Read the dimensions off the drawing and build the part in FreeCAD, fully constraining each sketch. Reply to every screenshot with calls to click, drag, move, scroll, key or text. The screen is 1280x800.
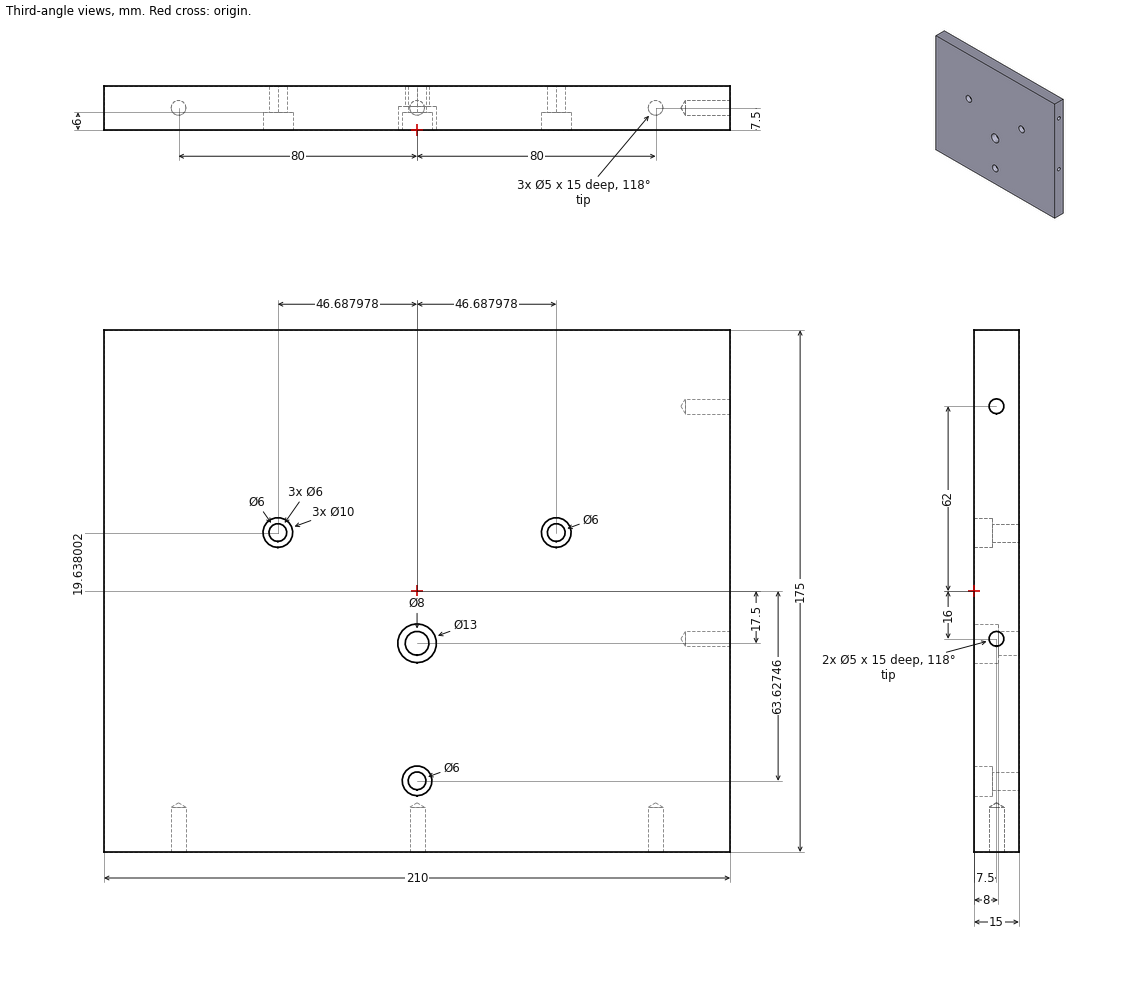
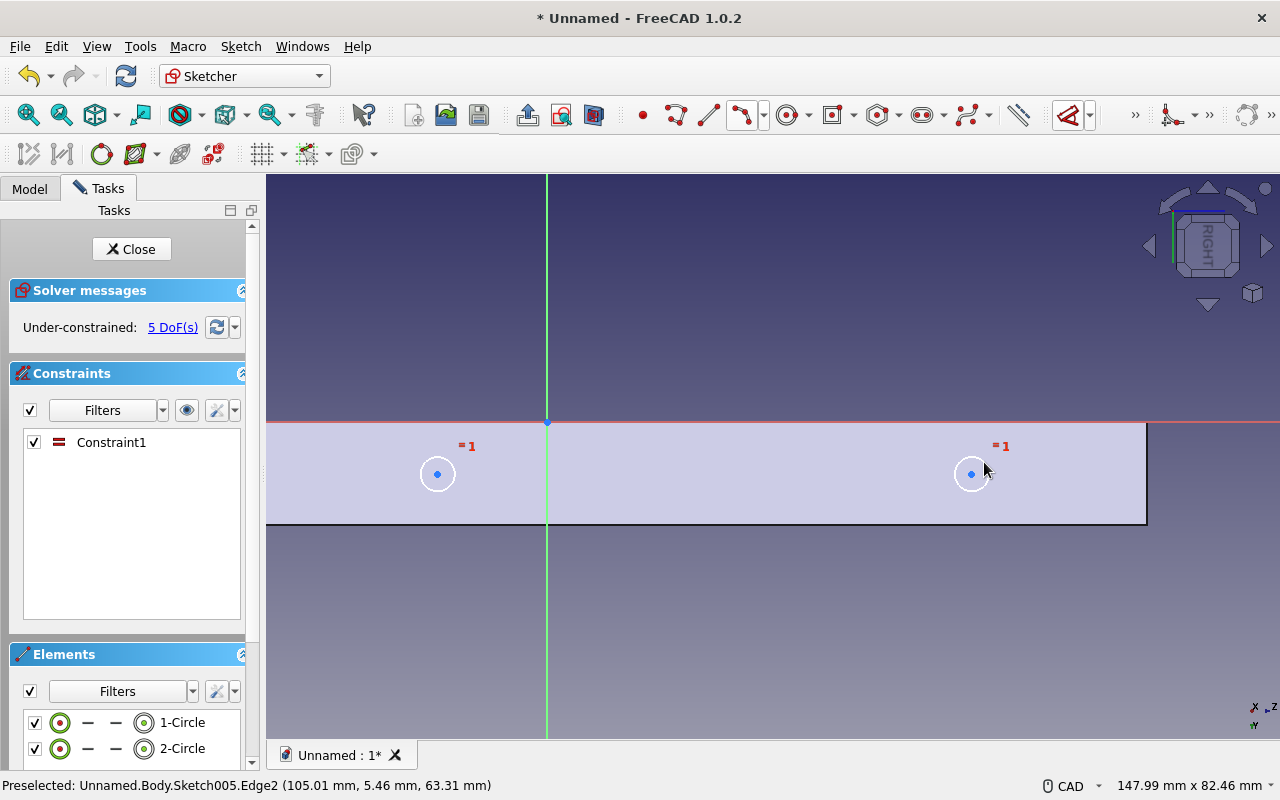
click(438, 474)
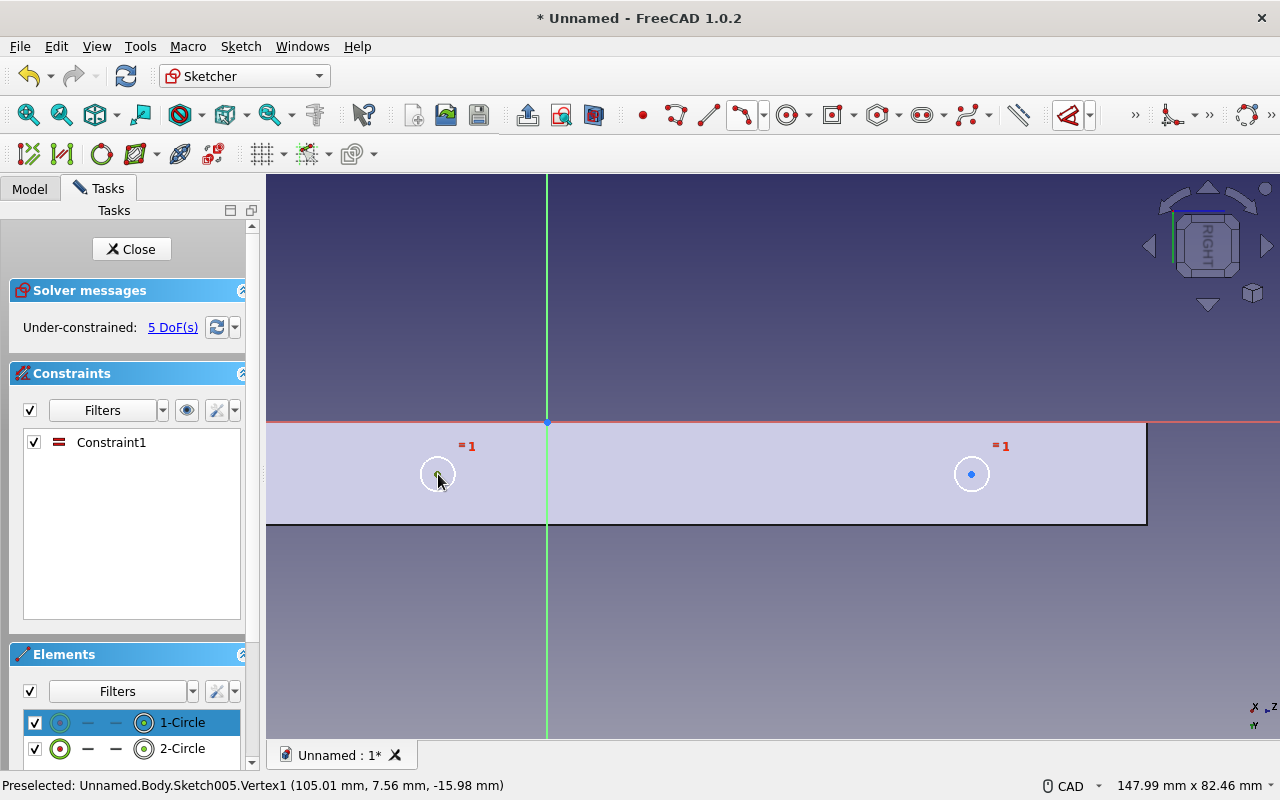
click(972, 474)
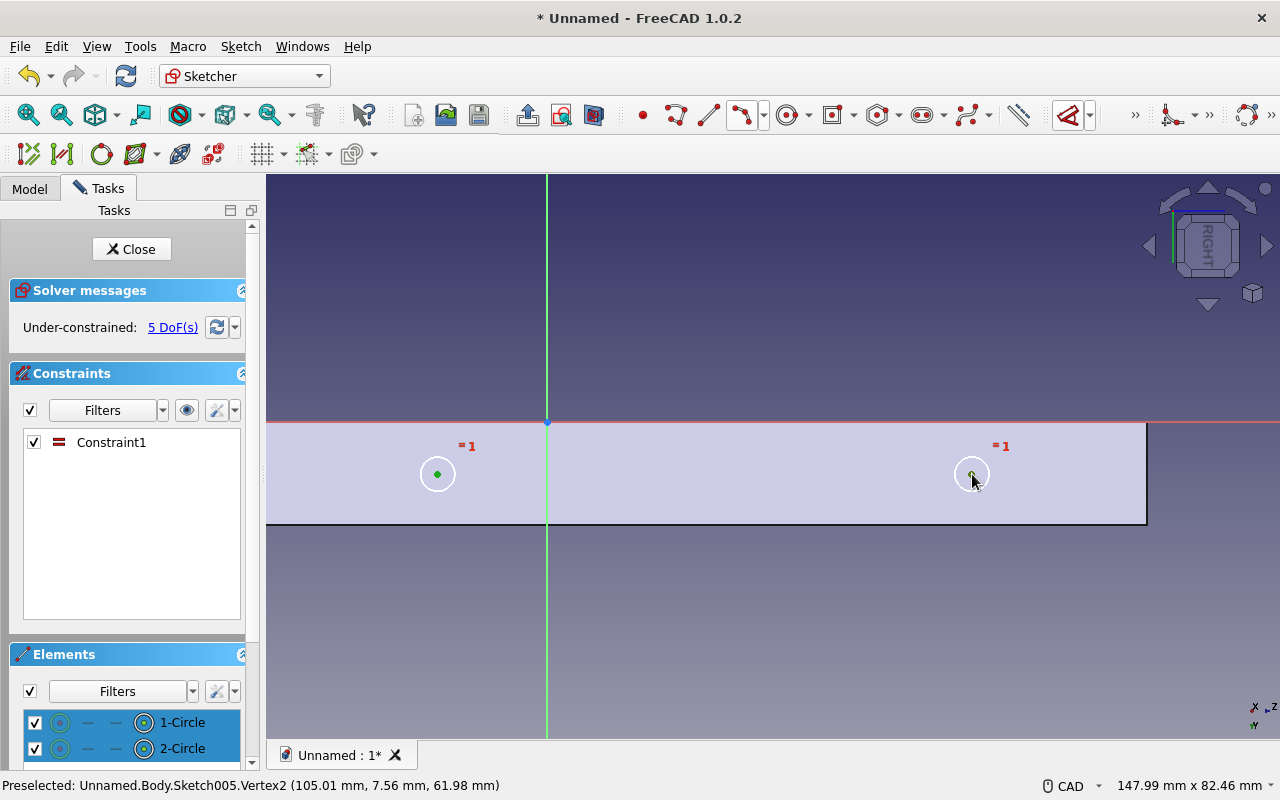
key(h)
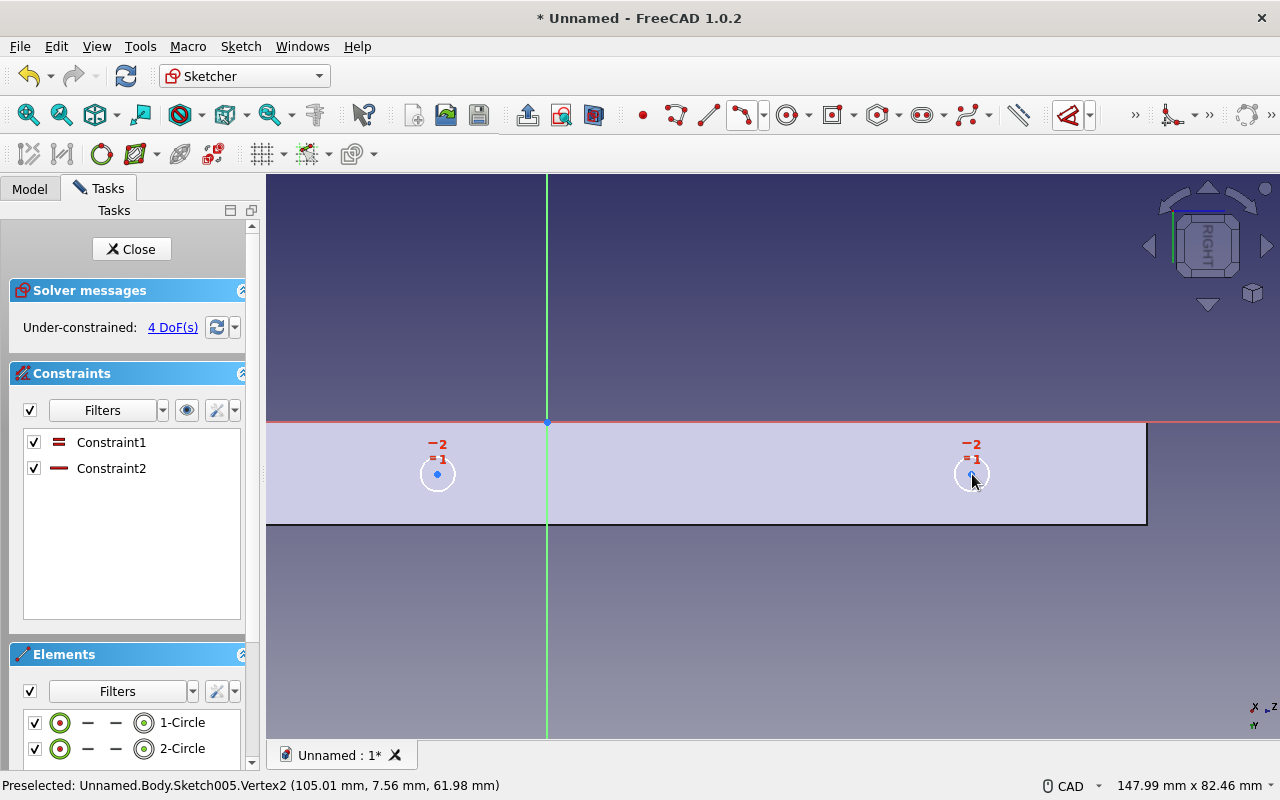
click(450, 462)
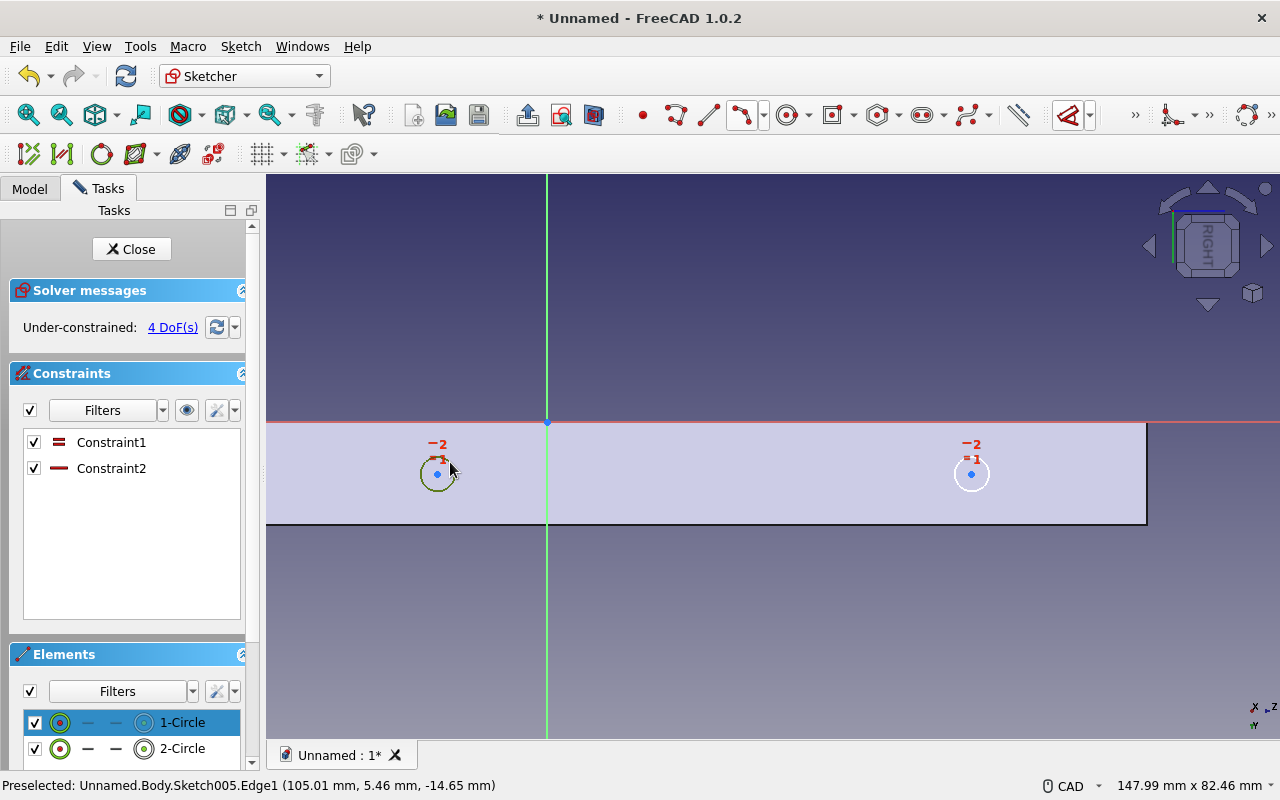
click(1090, 116)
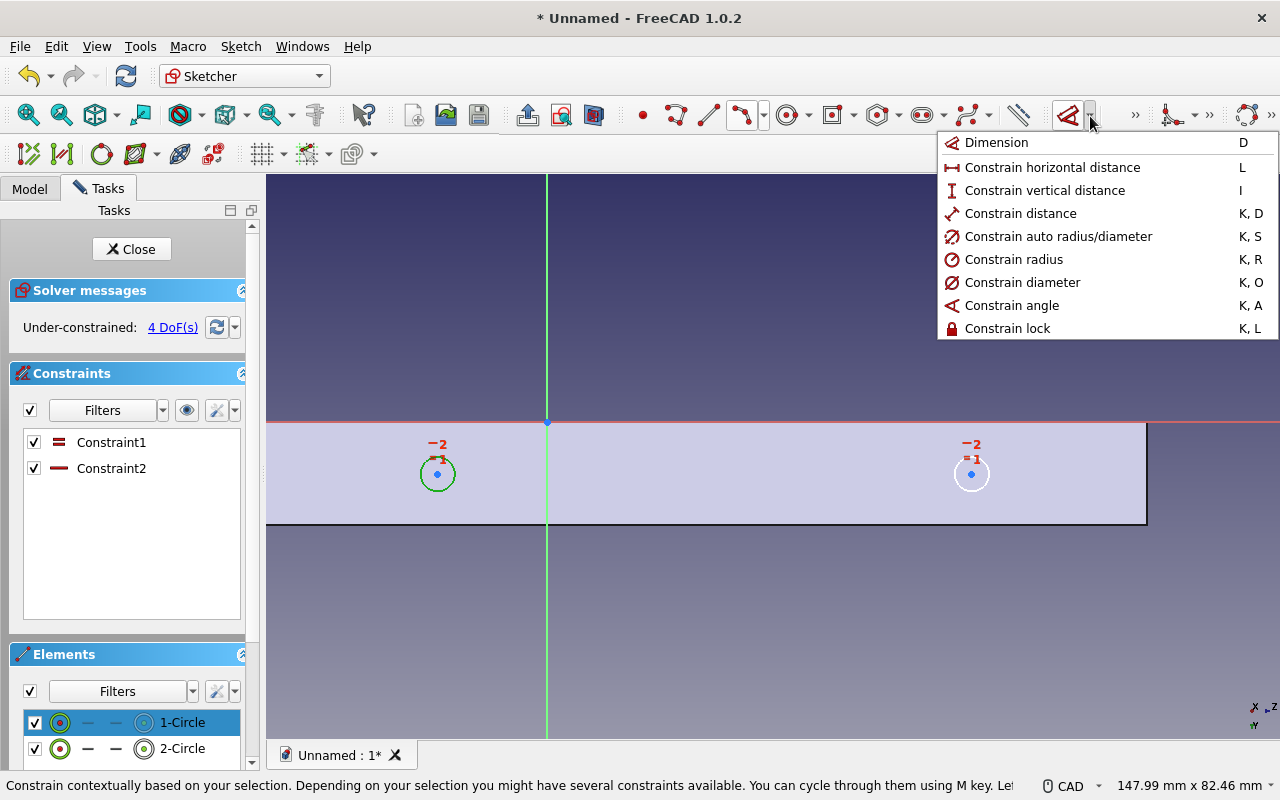
click(1108, 282)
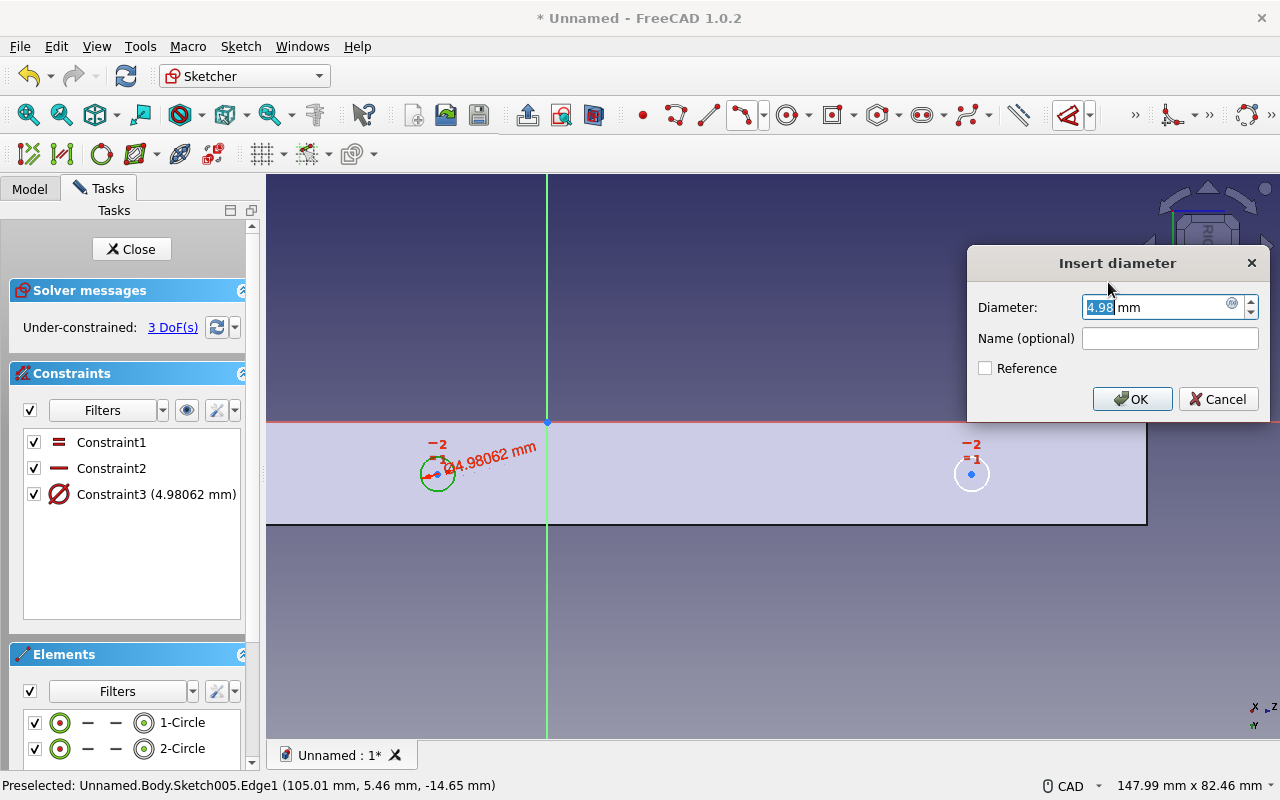
text(5)
key(Return)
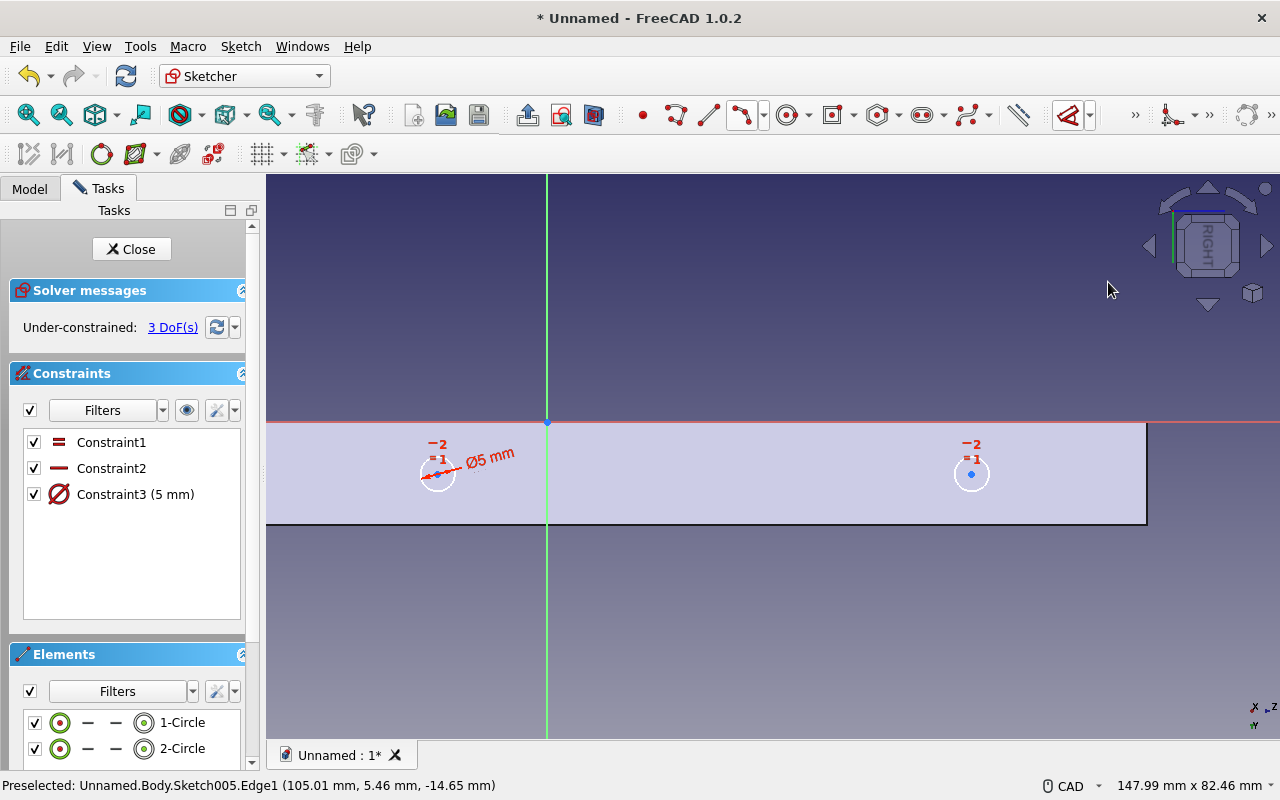
click(438, 474)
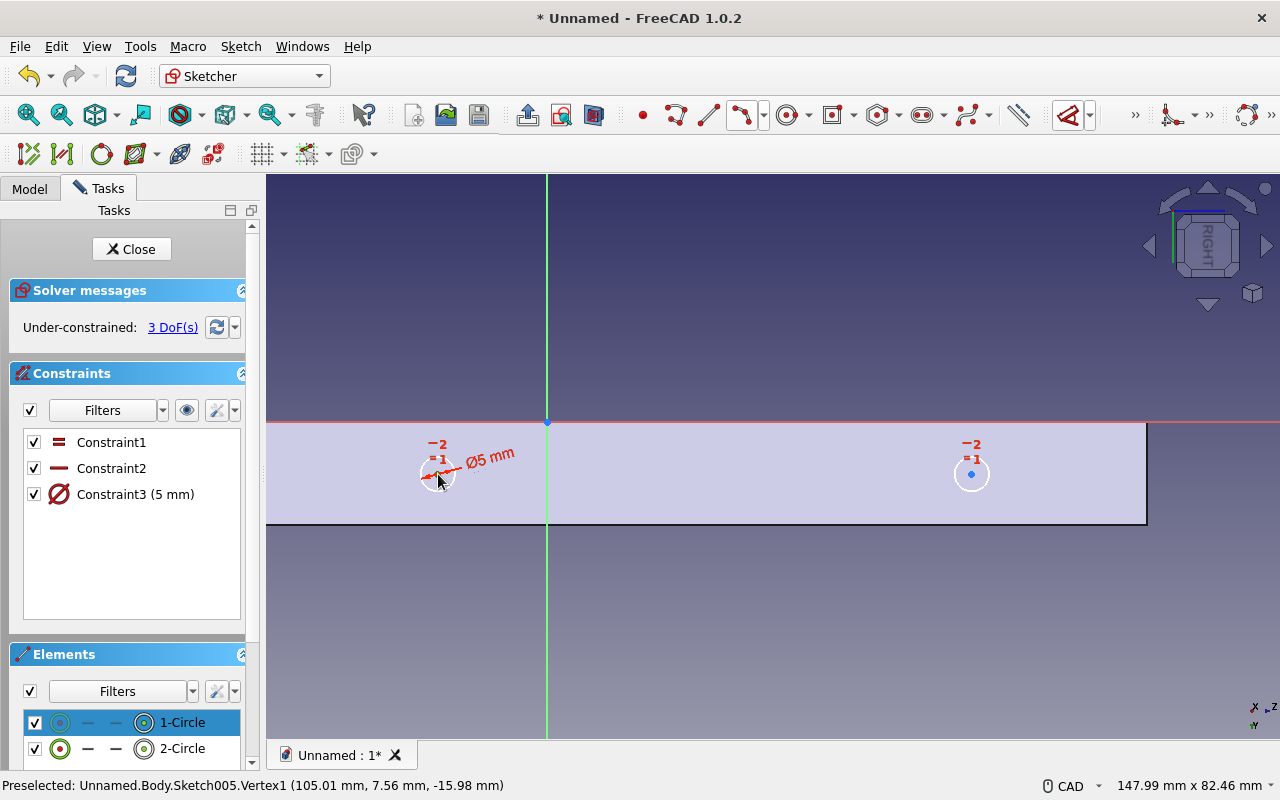
key(l)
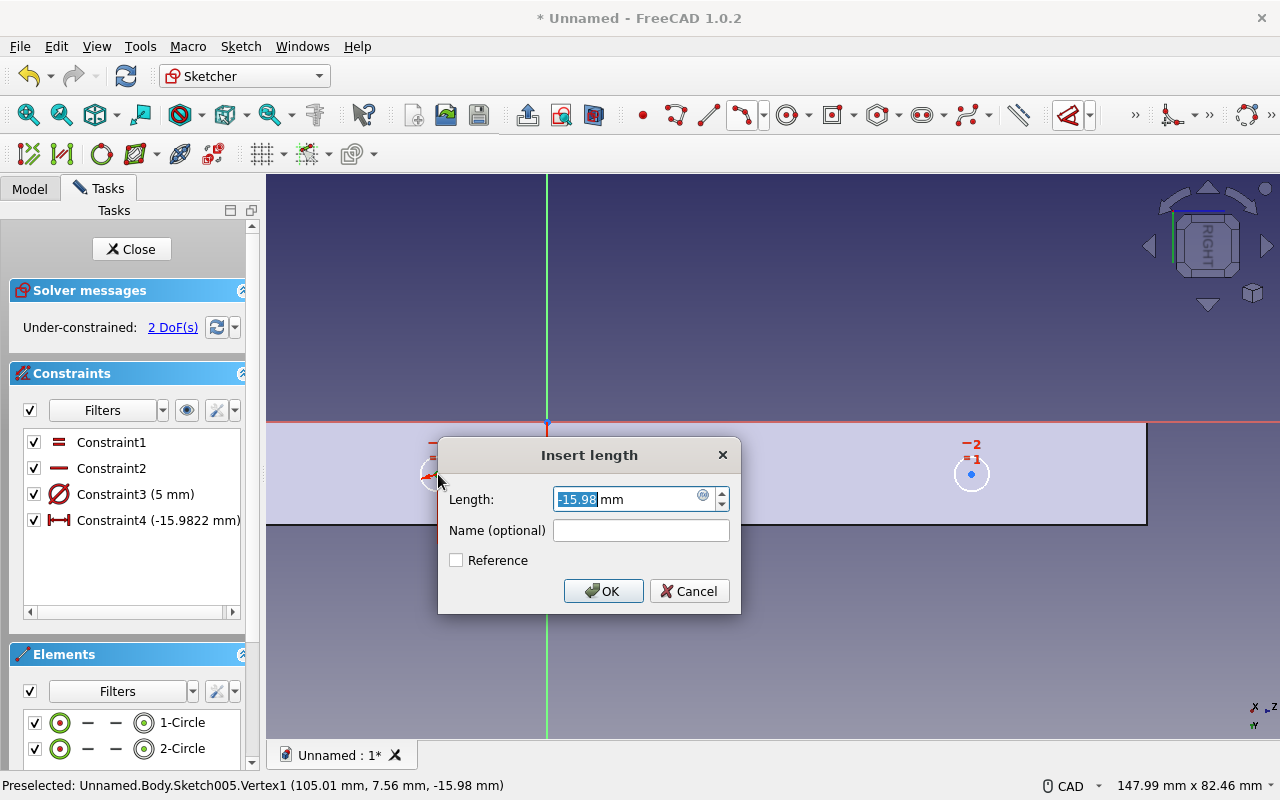
text(-16)
key(Return)